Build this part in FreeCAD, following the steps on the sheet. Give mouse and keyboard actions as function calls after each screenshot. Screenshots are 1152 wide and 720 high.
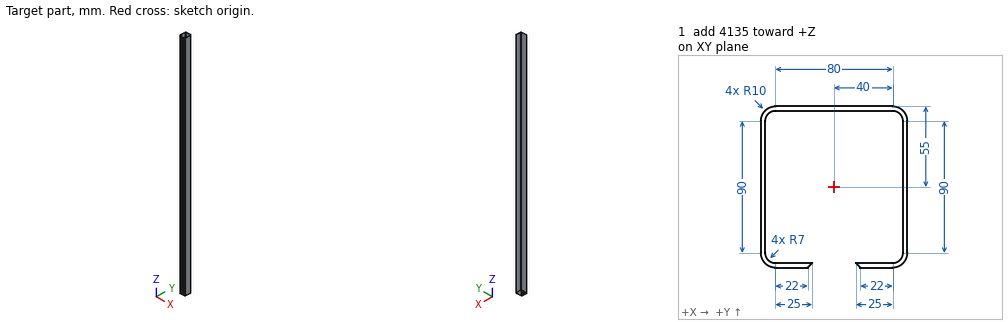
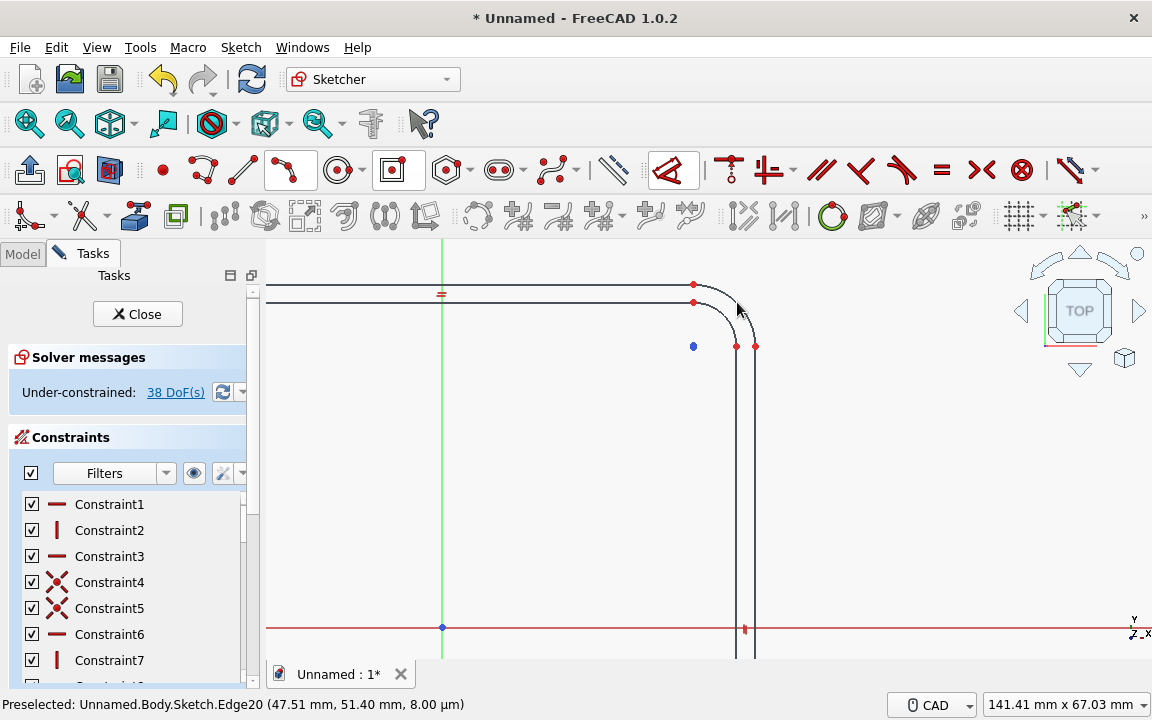
click(542, 285)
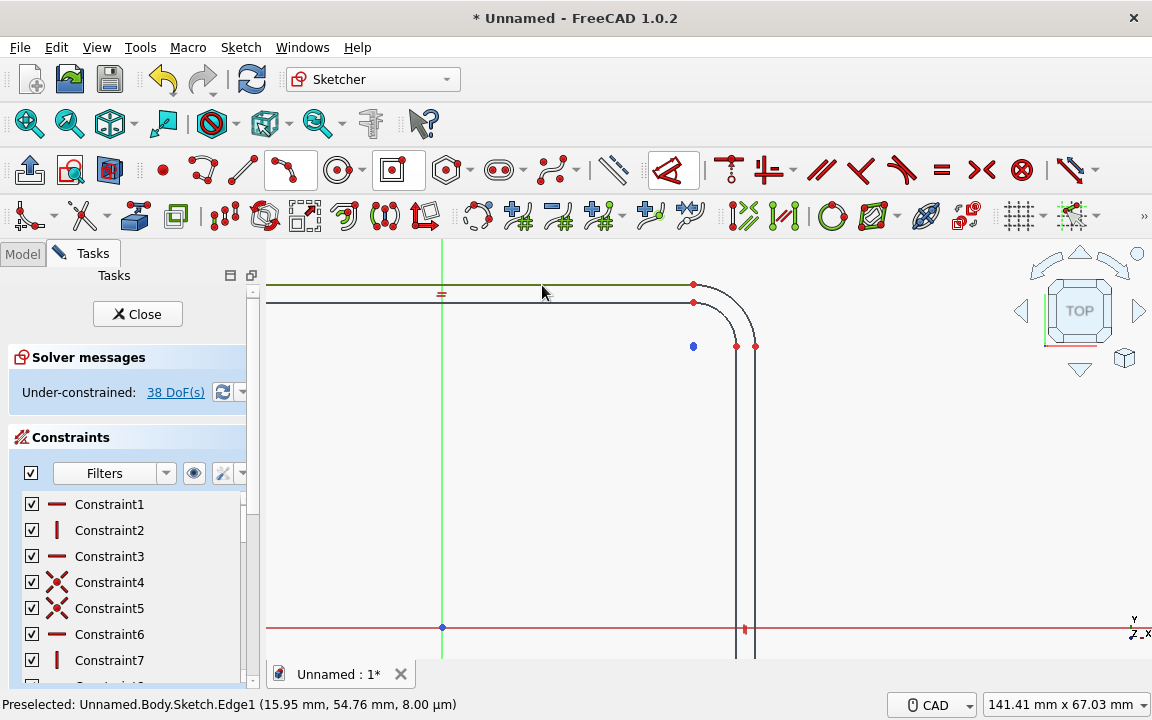
scroll(756, 345, down, 5)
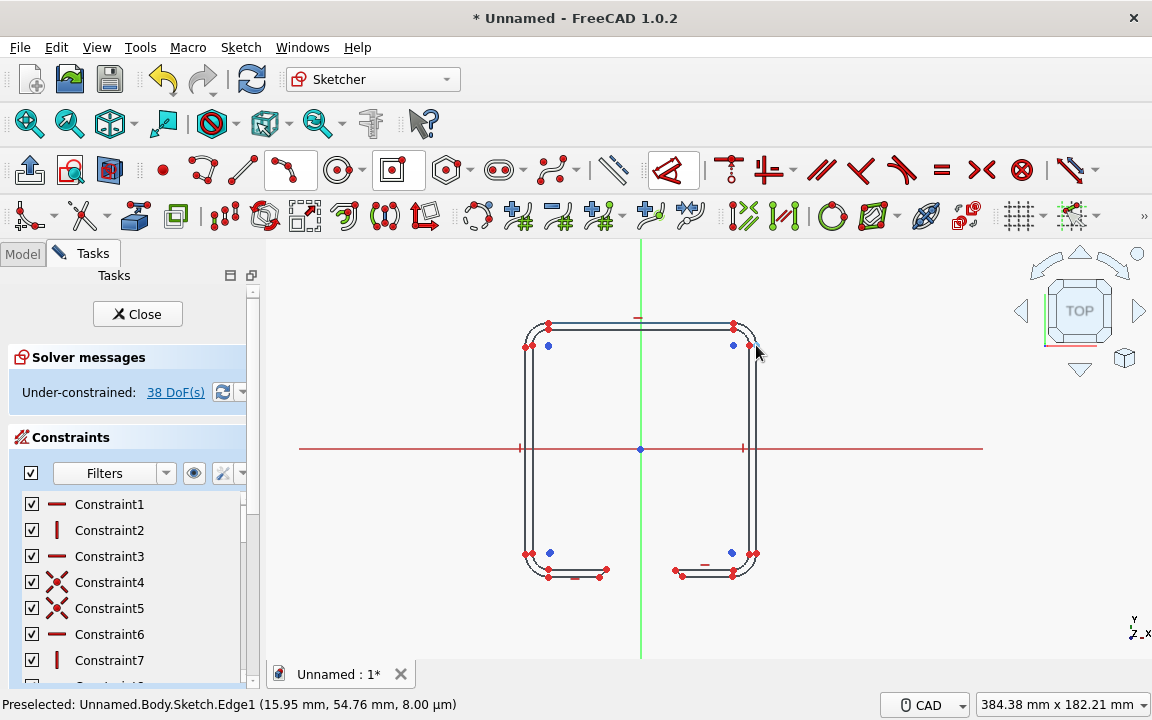
scroll(538, 326, up, 4)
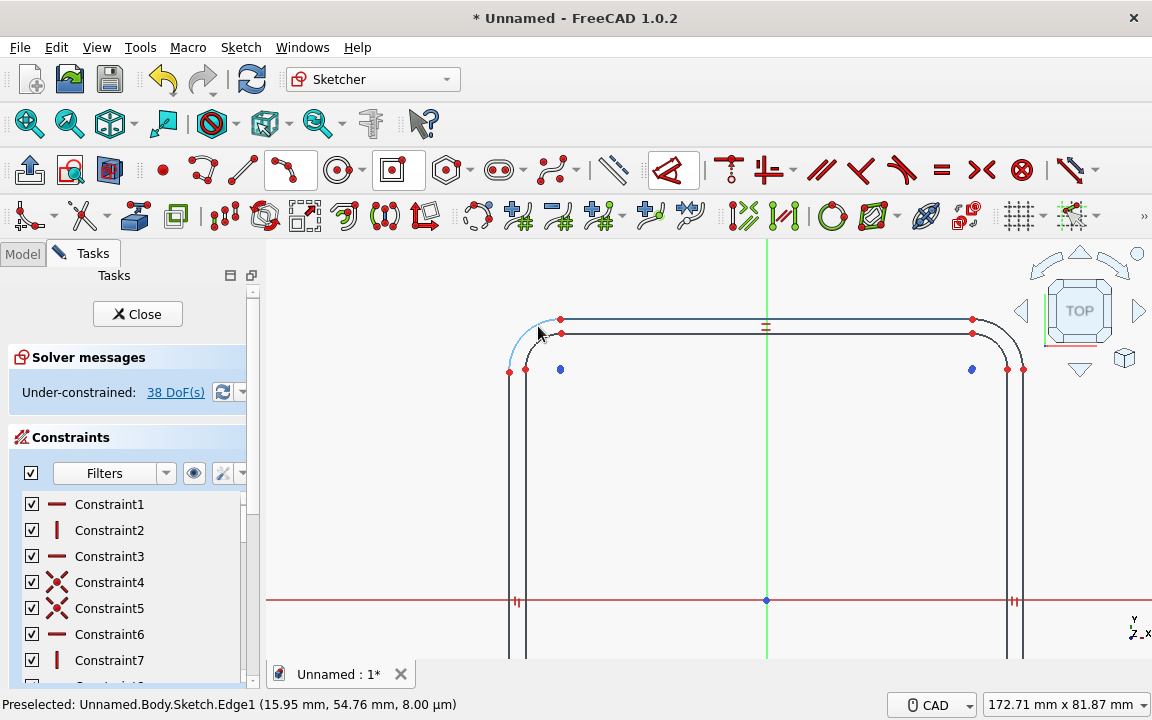
click(537, 325)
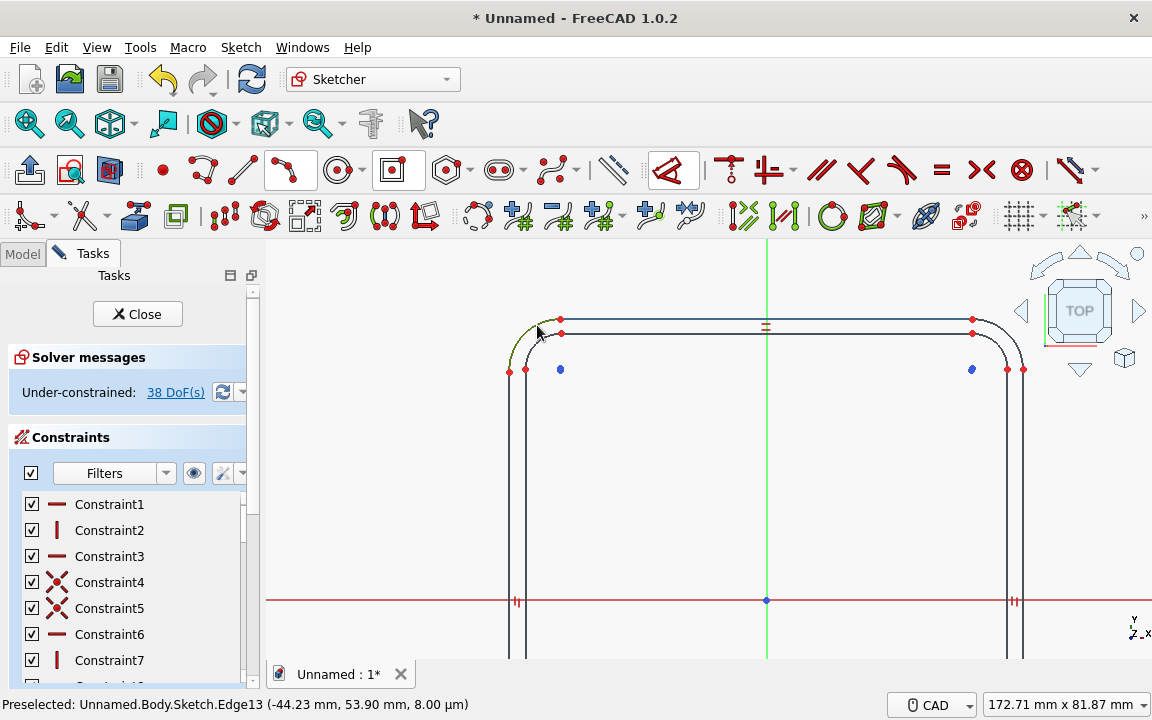
click(902, 170)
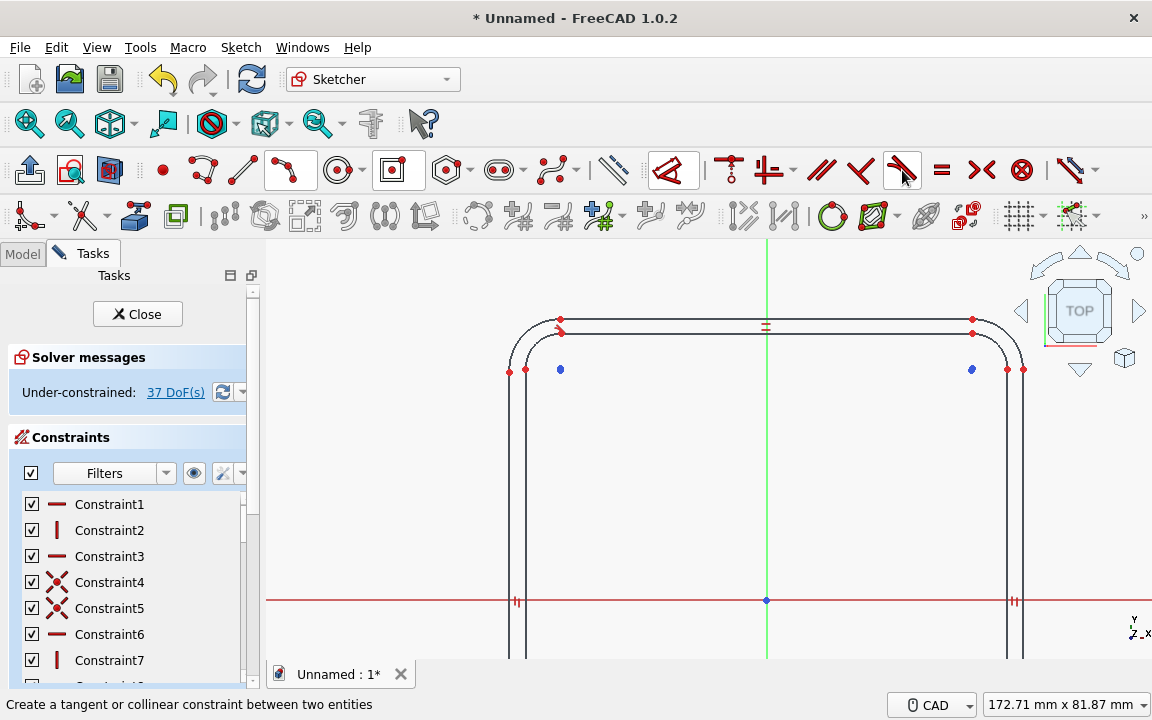
click(849, 319)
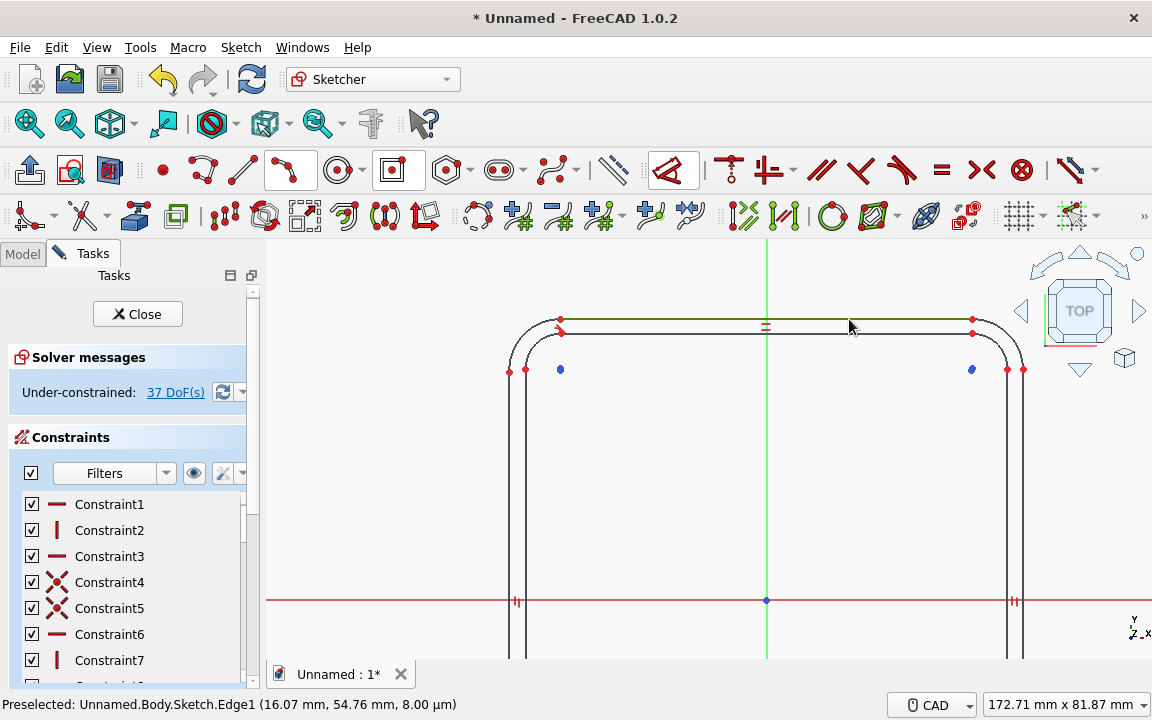
scroll(538, 326, down, 4)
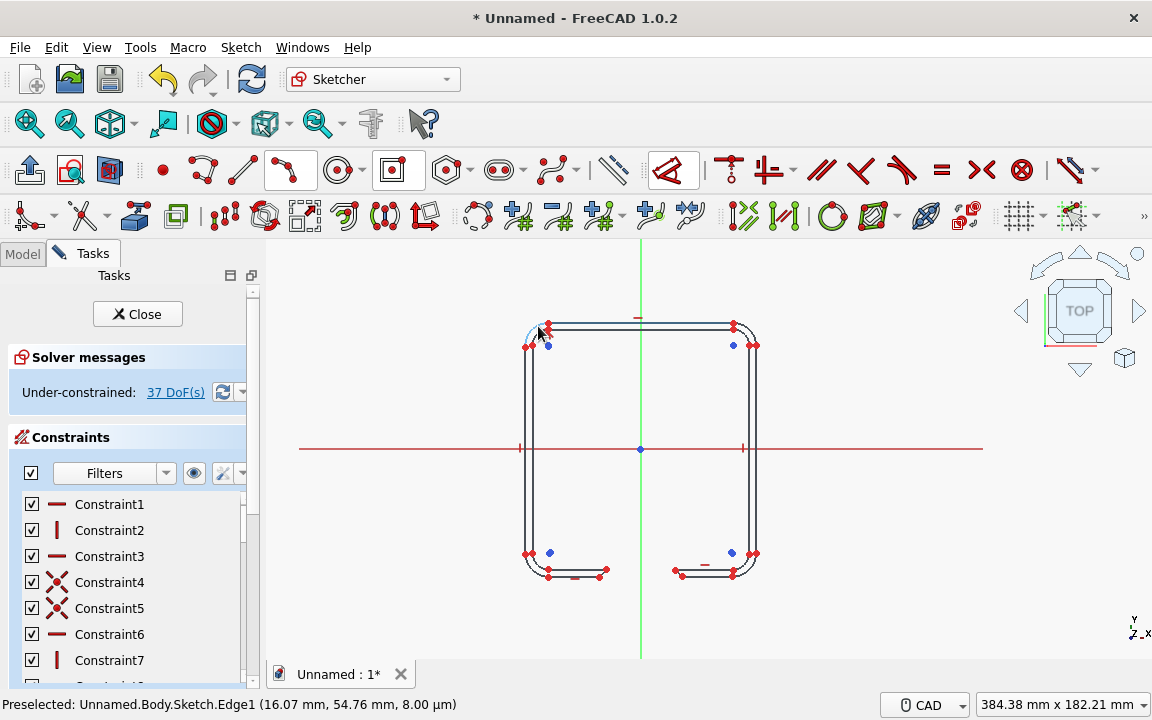
scroll(754, 335, up, 4)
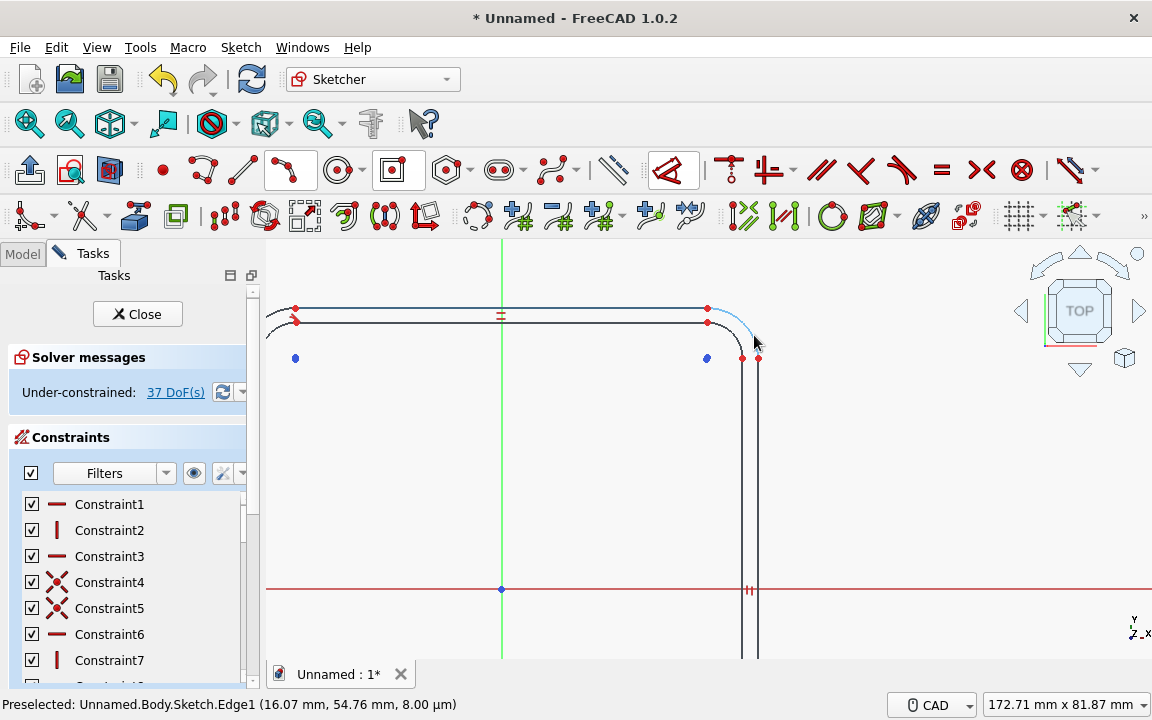
click(752, 336)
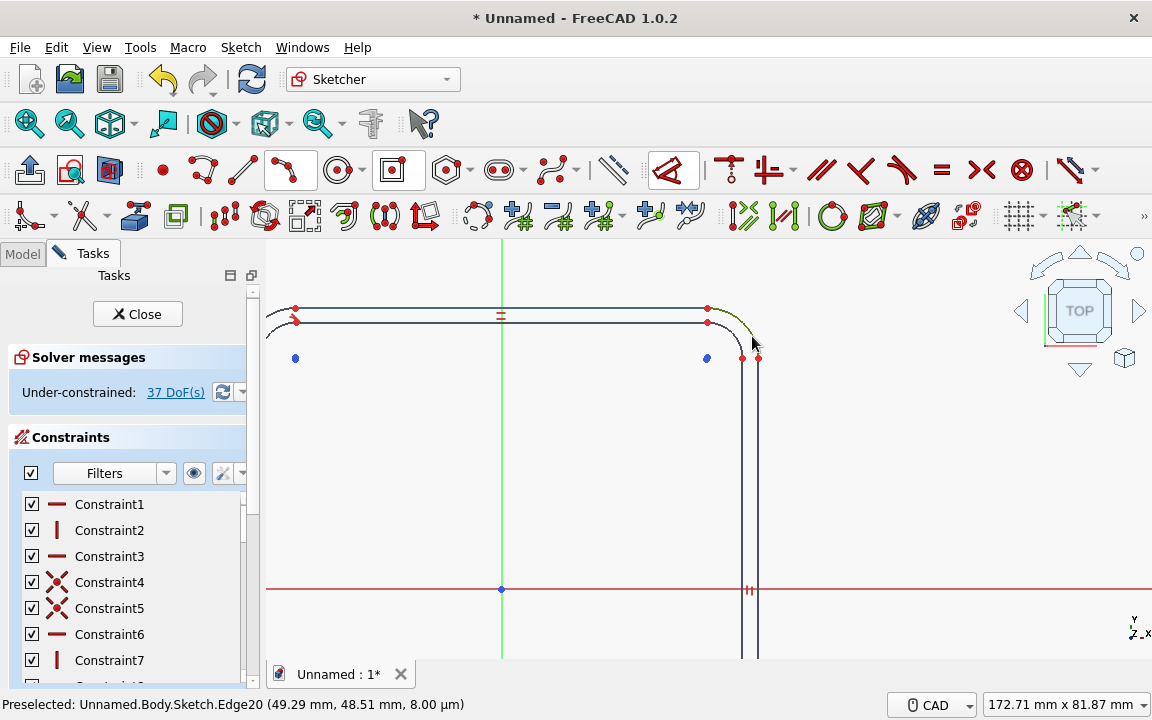
click(902, 170)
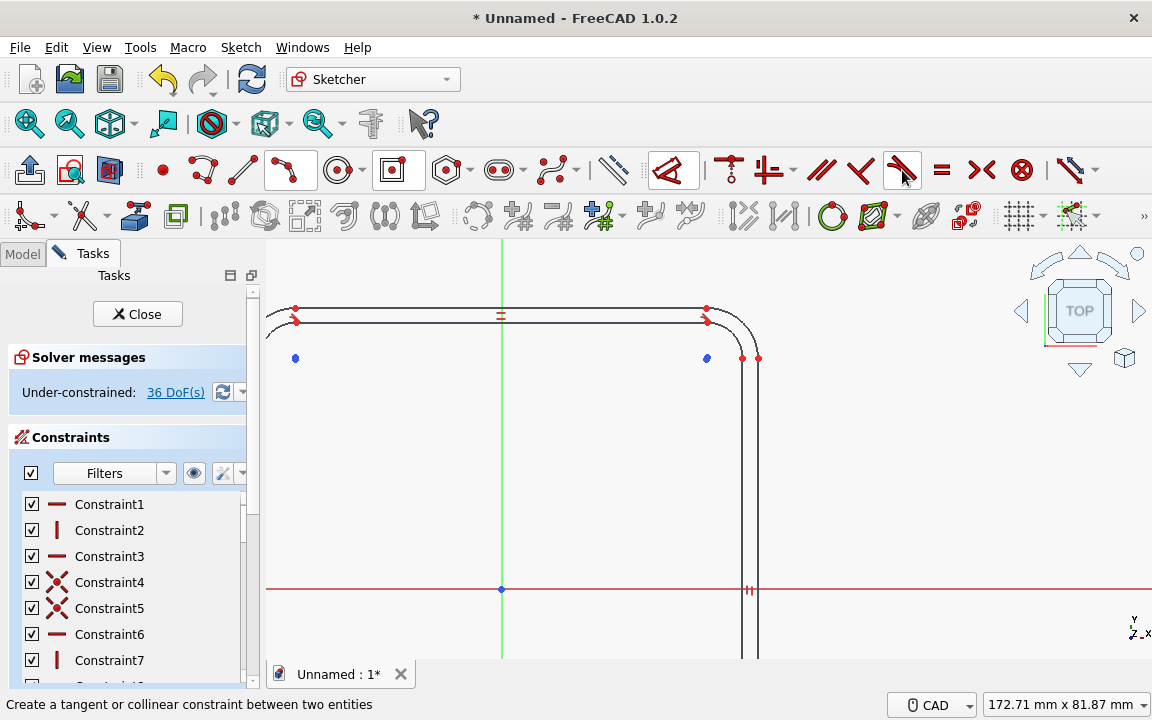
scroll(754, 335, down, 4)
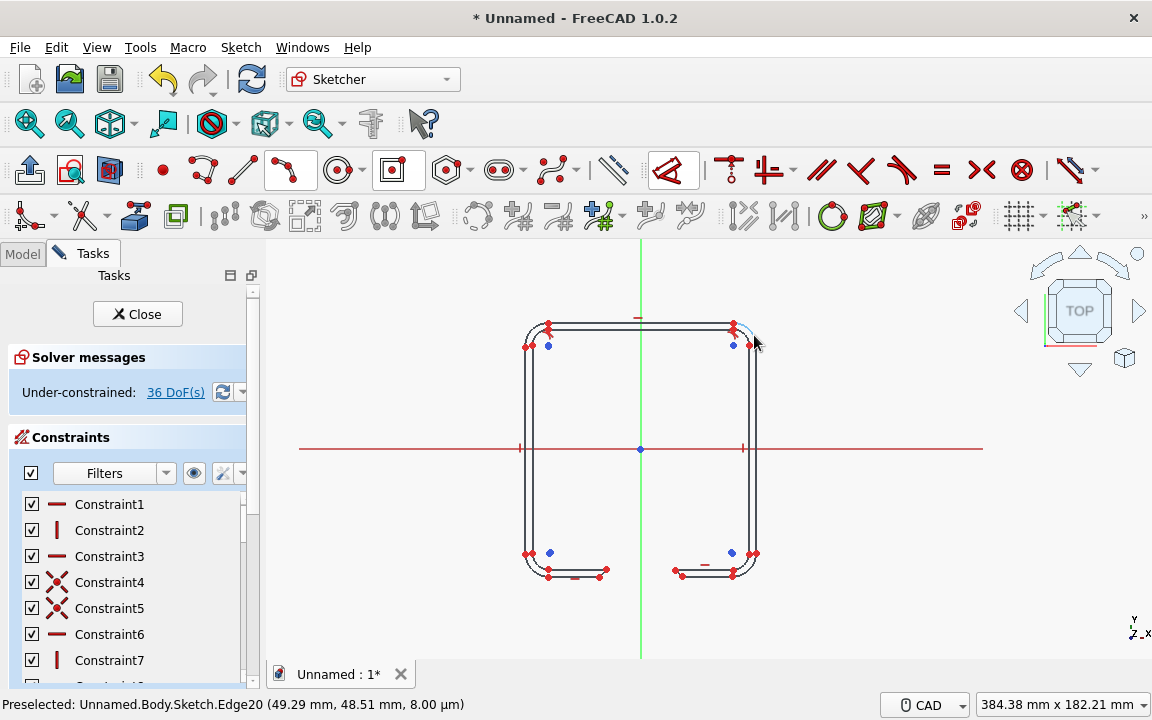
scroll(525, 409, up, 4)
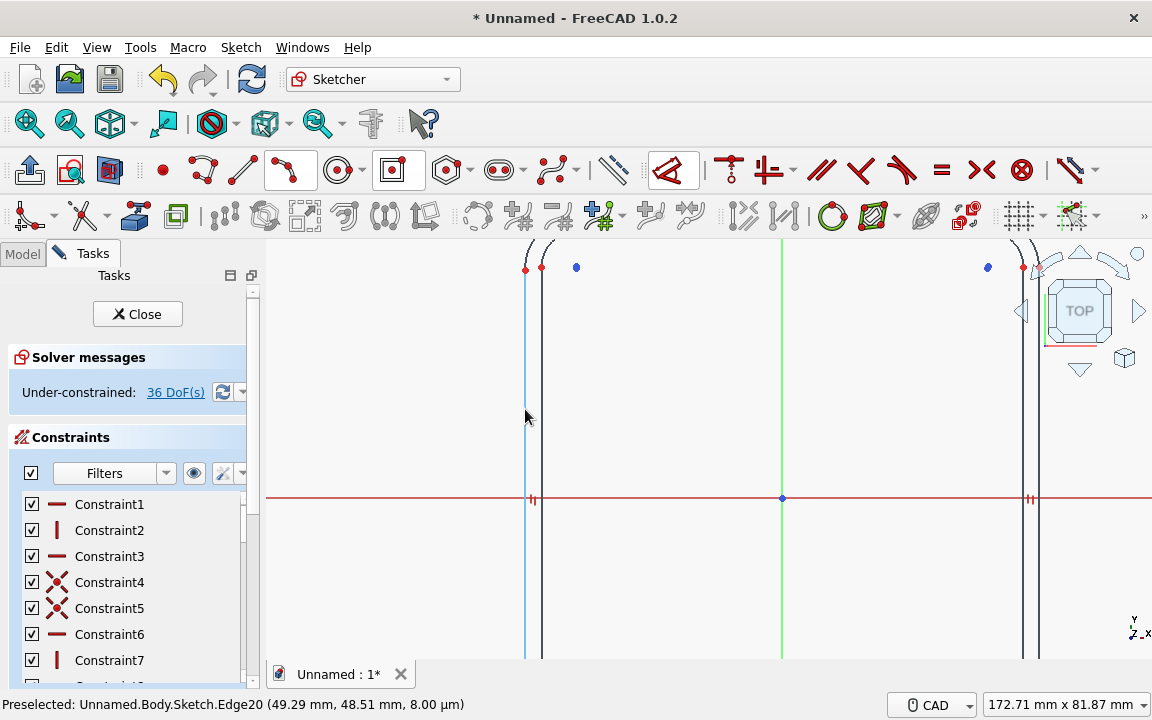
click(525, 409)